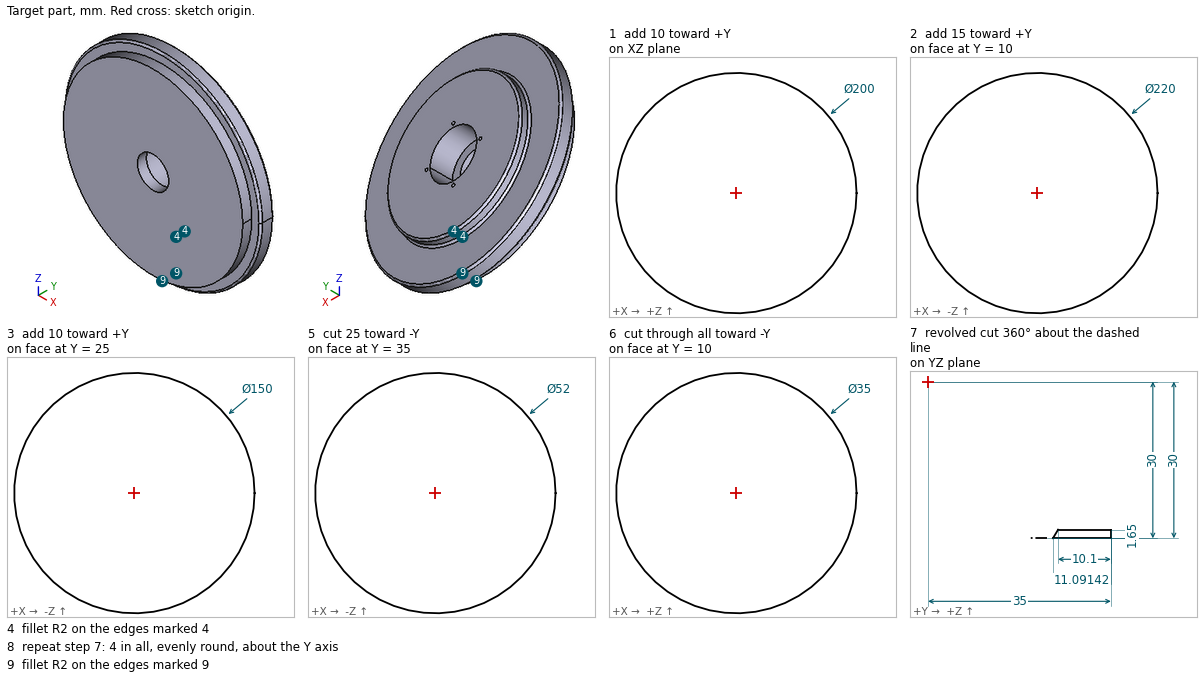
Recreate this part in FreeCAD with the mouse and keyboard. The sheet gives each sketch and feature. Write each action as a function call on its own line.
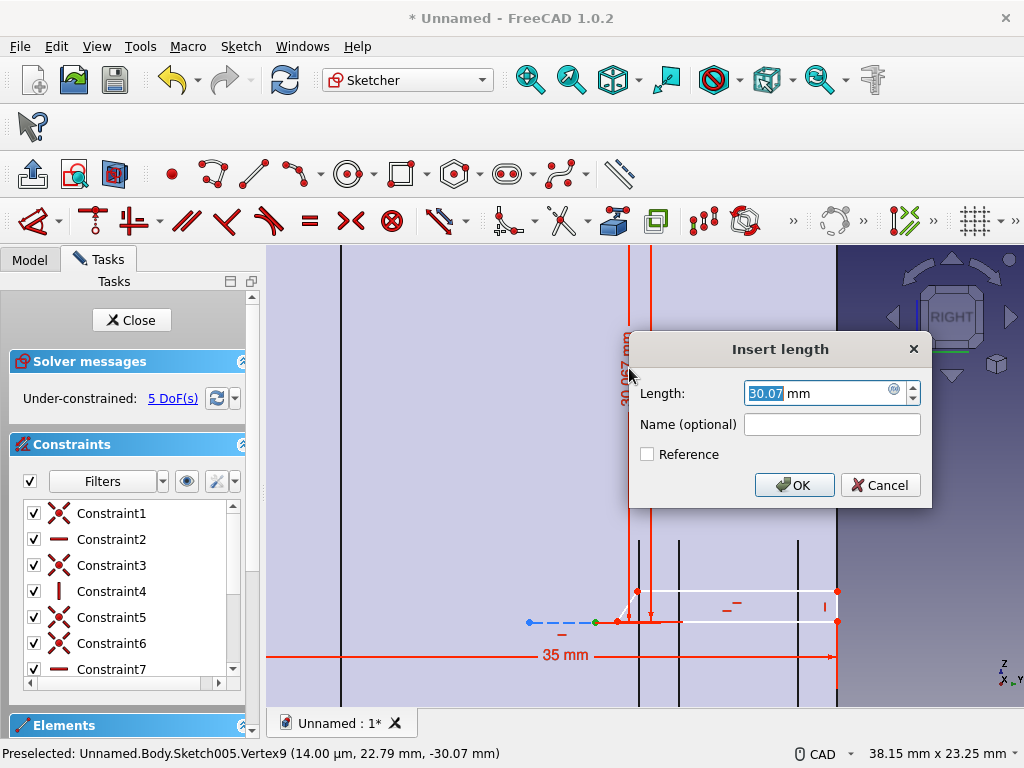
text(30)
key(Return)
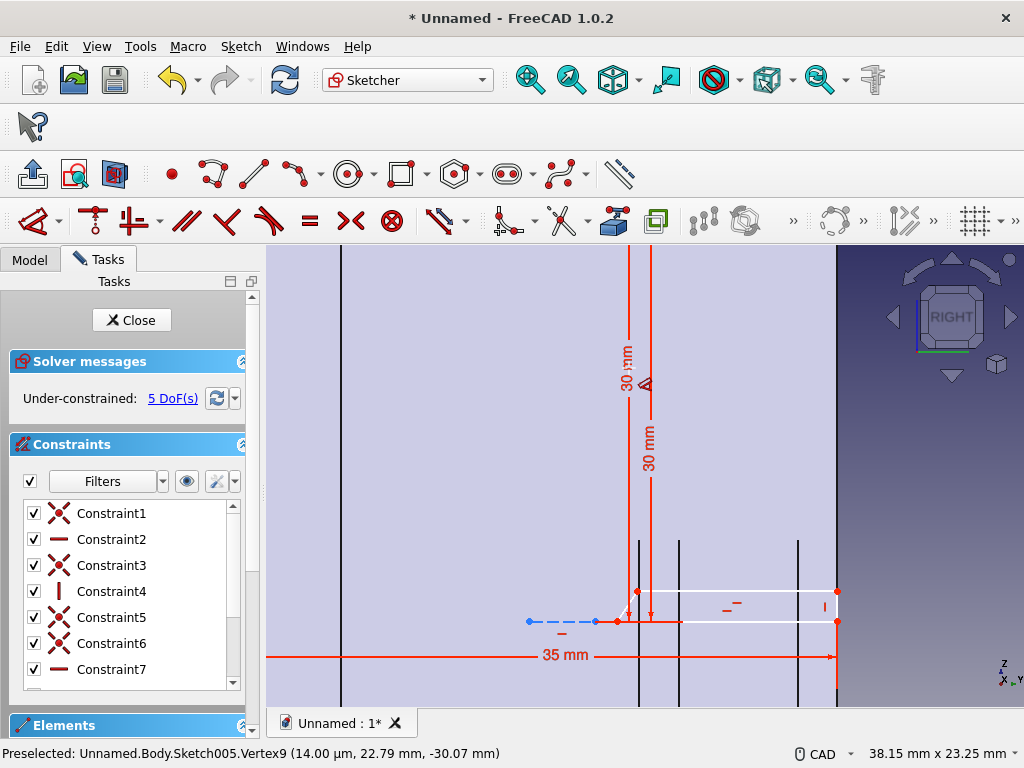
scroll(837, 613, up, 3)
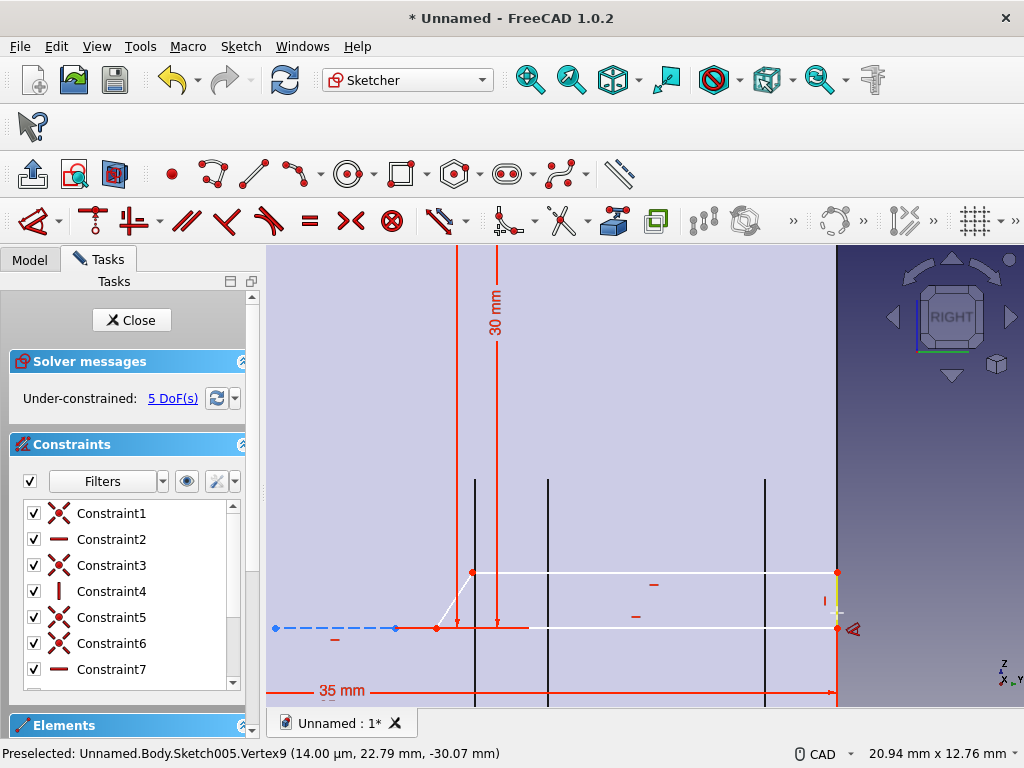
click(837, 612)
click(803, 600)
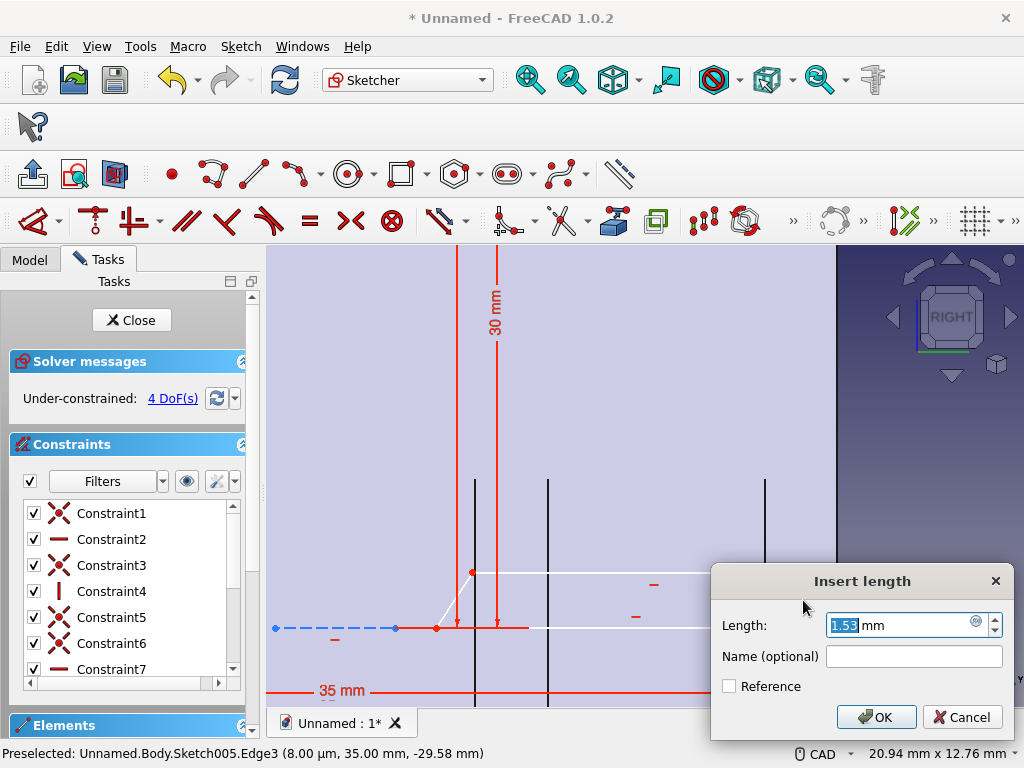
text(1.65)
key(Return)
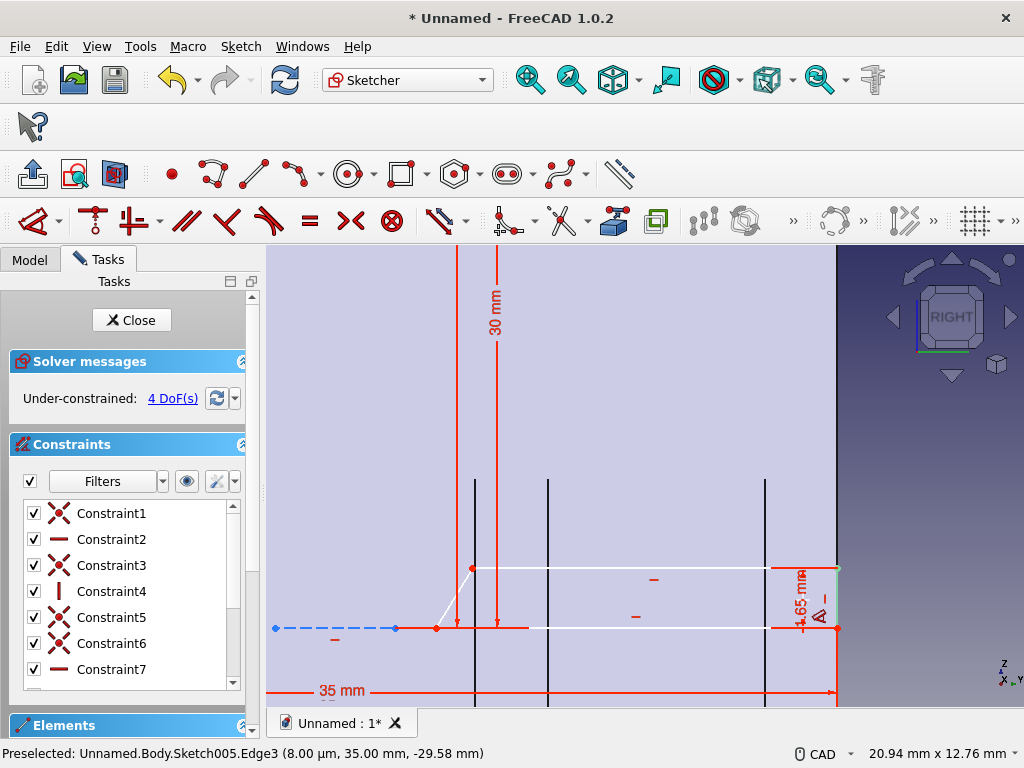
scroll(699, 604, down, 7)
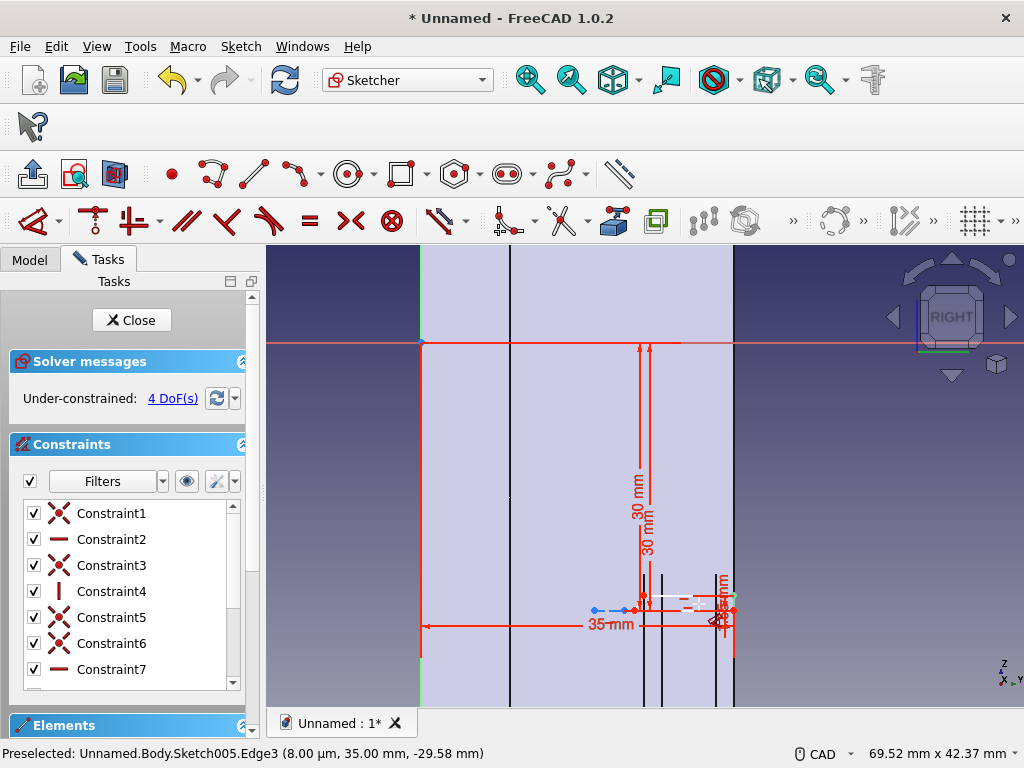
click(707, 596)
click(689, 630)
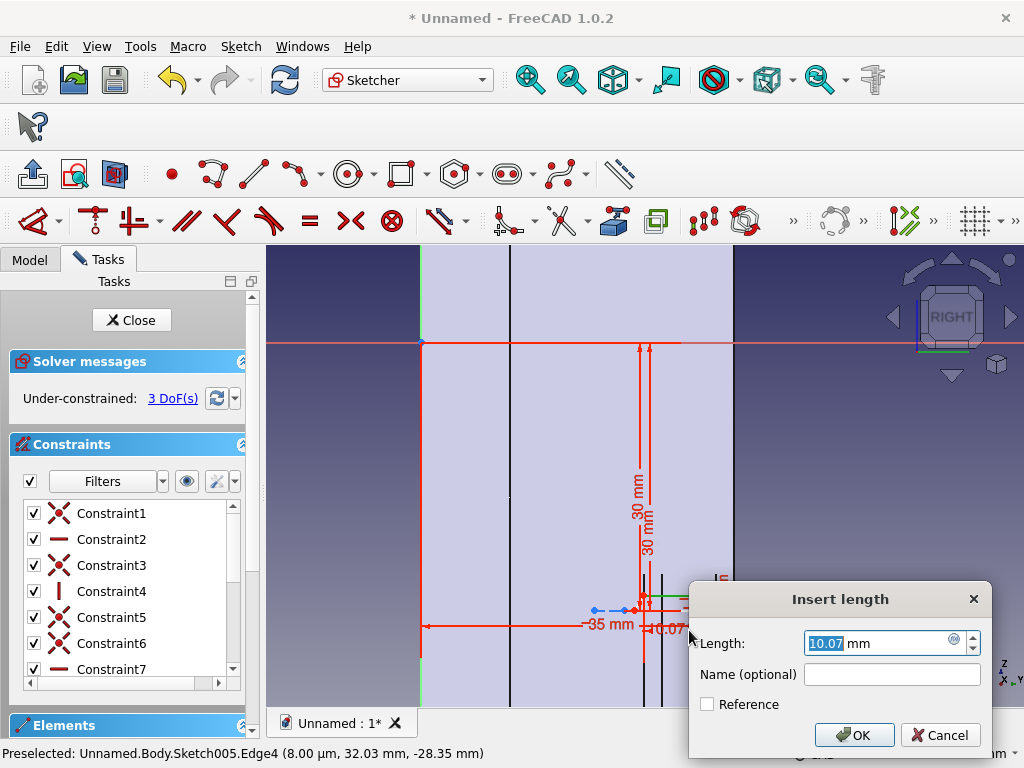
text(10.1)
key(Return)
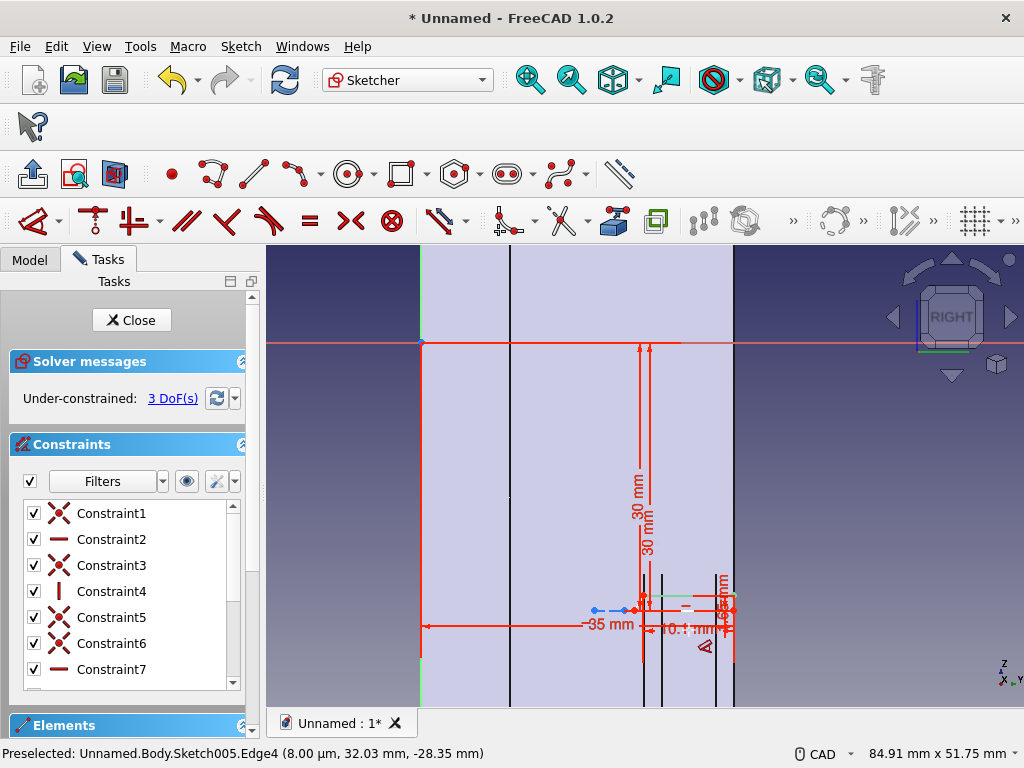
click(664, 611)
click(684, 577)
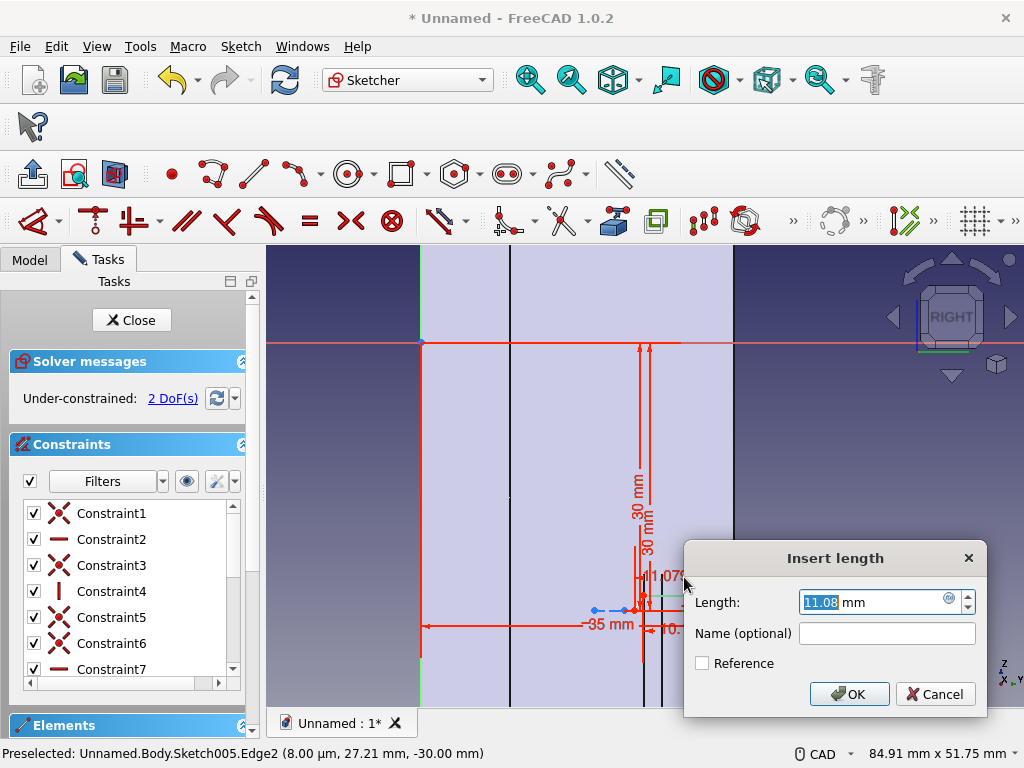
text(11.09142)
key(Return)
key(Escape)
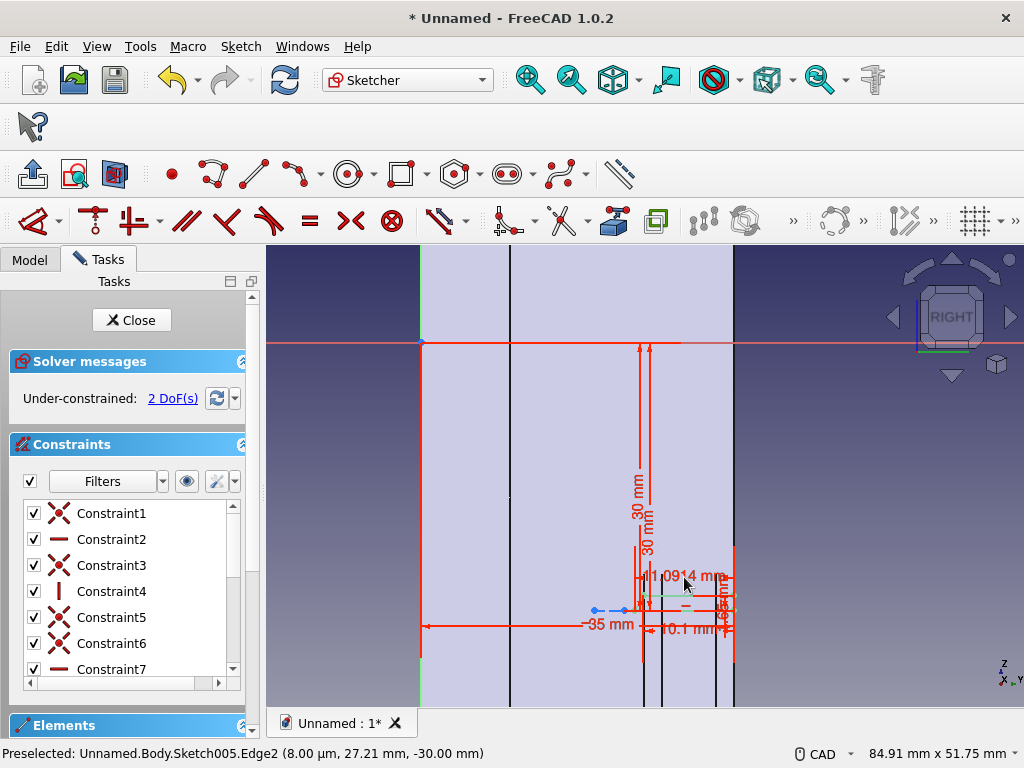
click(132, 320)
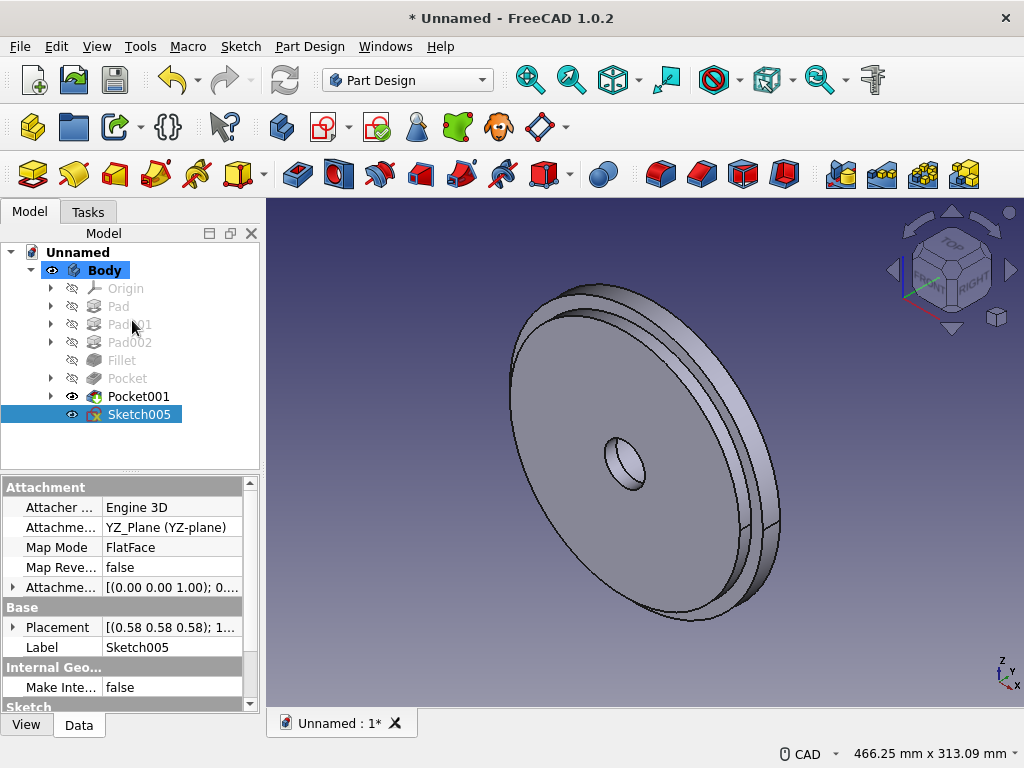
click(380, 174)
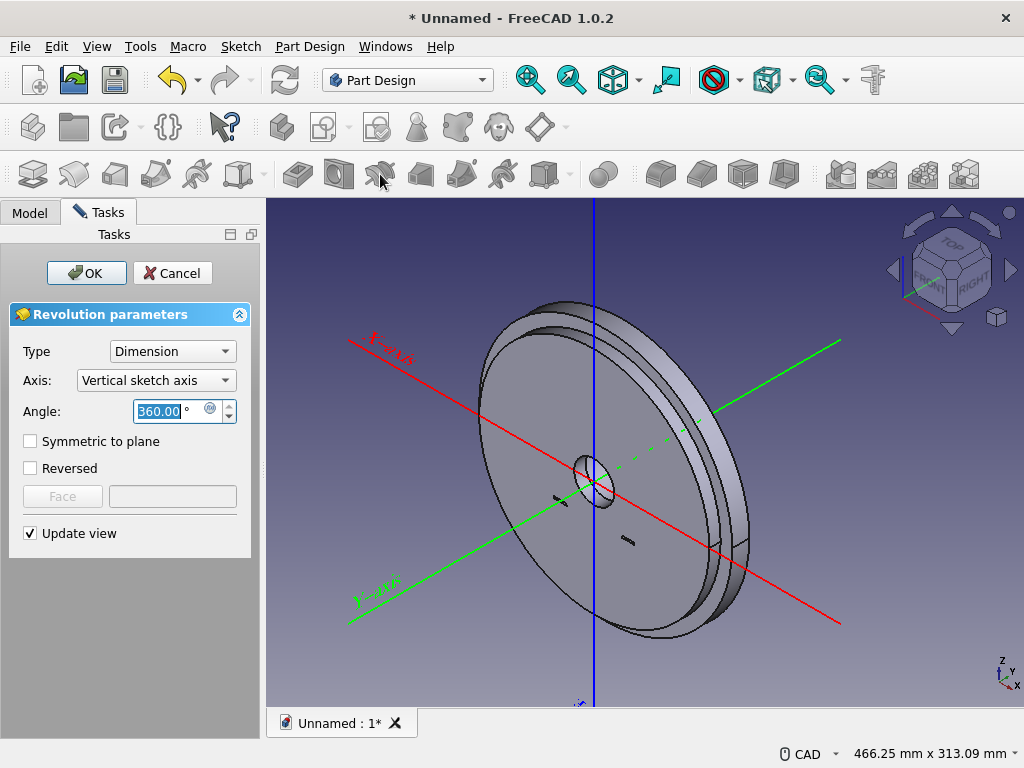
click(157, 380)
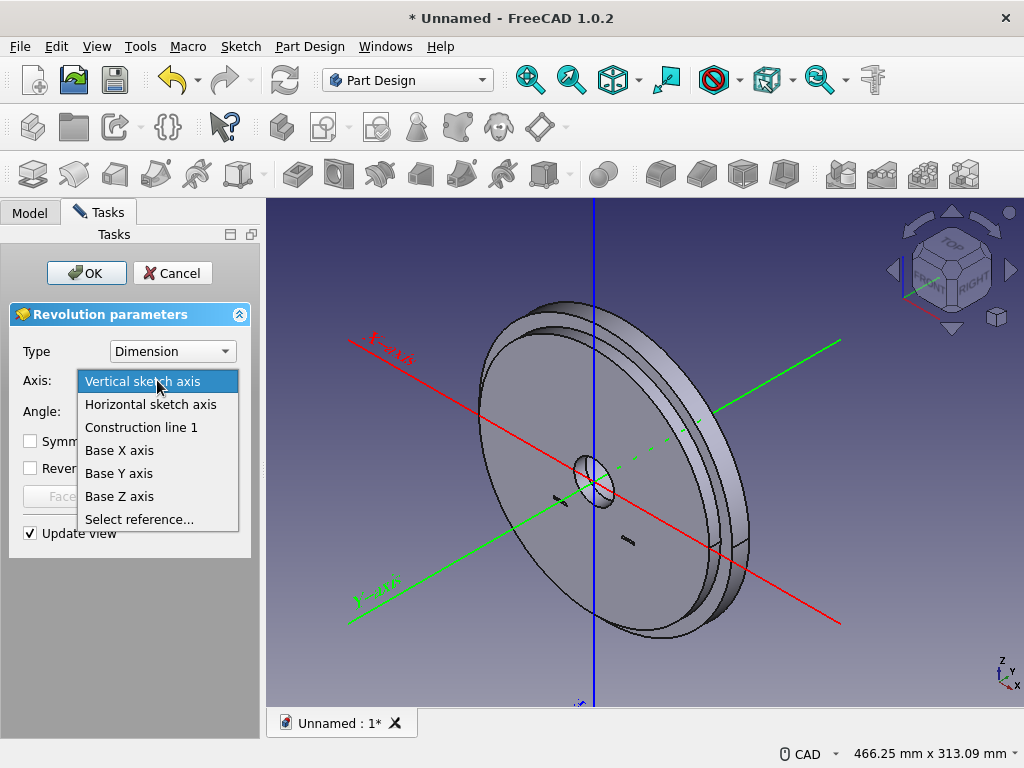
click(156, 428)